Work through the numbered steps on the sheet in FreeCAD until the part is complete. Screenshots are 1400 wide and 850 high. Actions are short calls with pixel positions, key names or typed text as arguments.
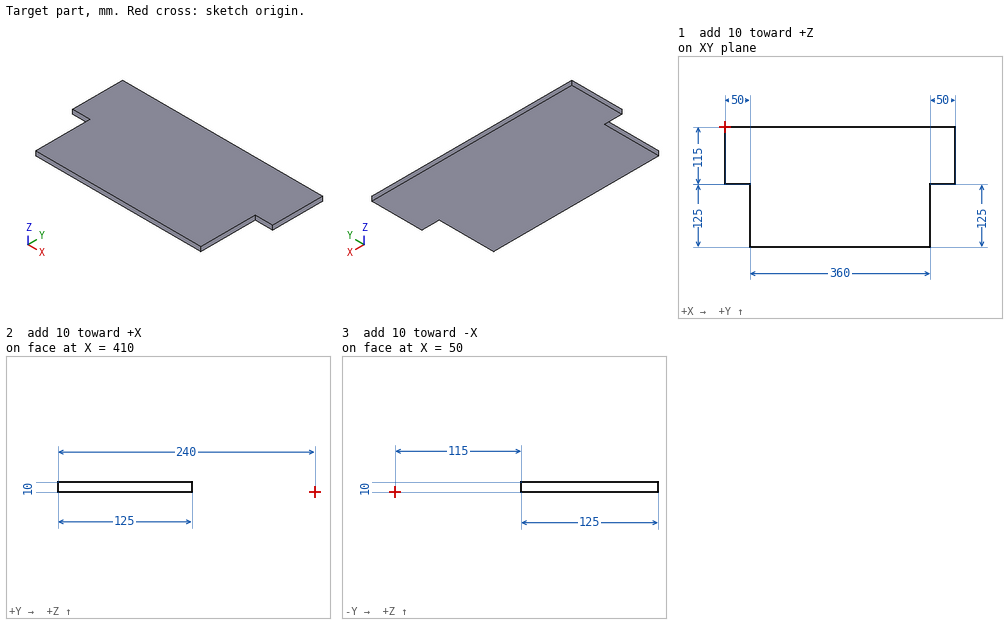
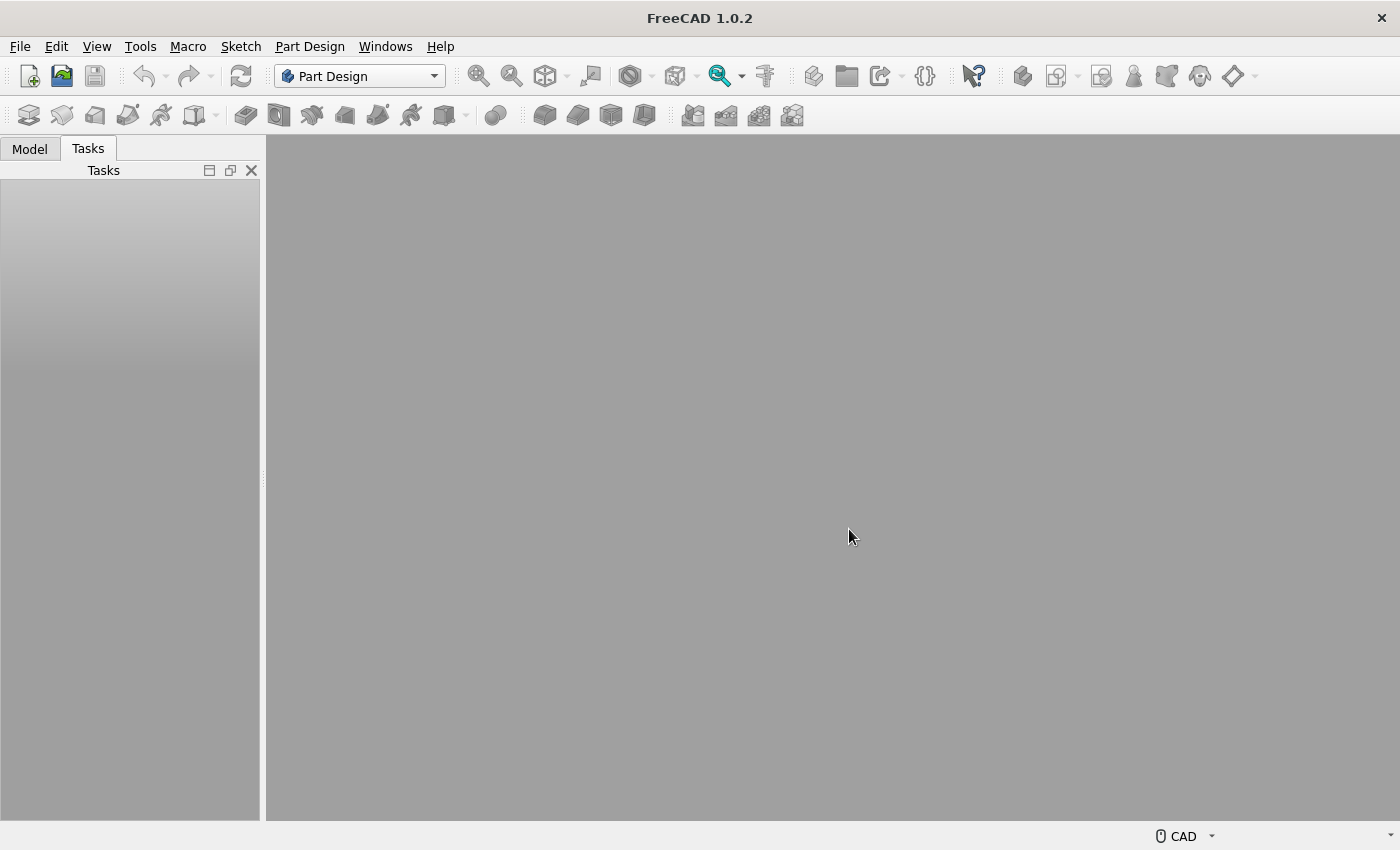
click(29, 76)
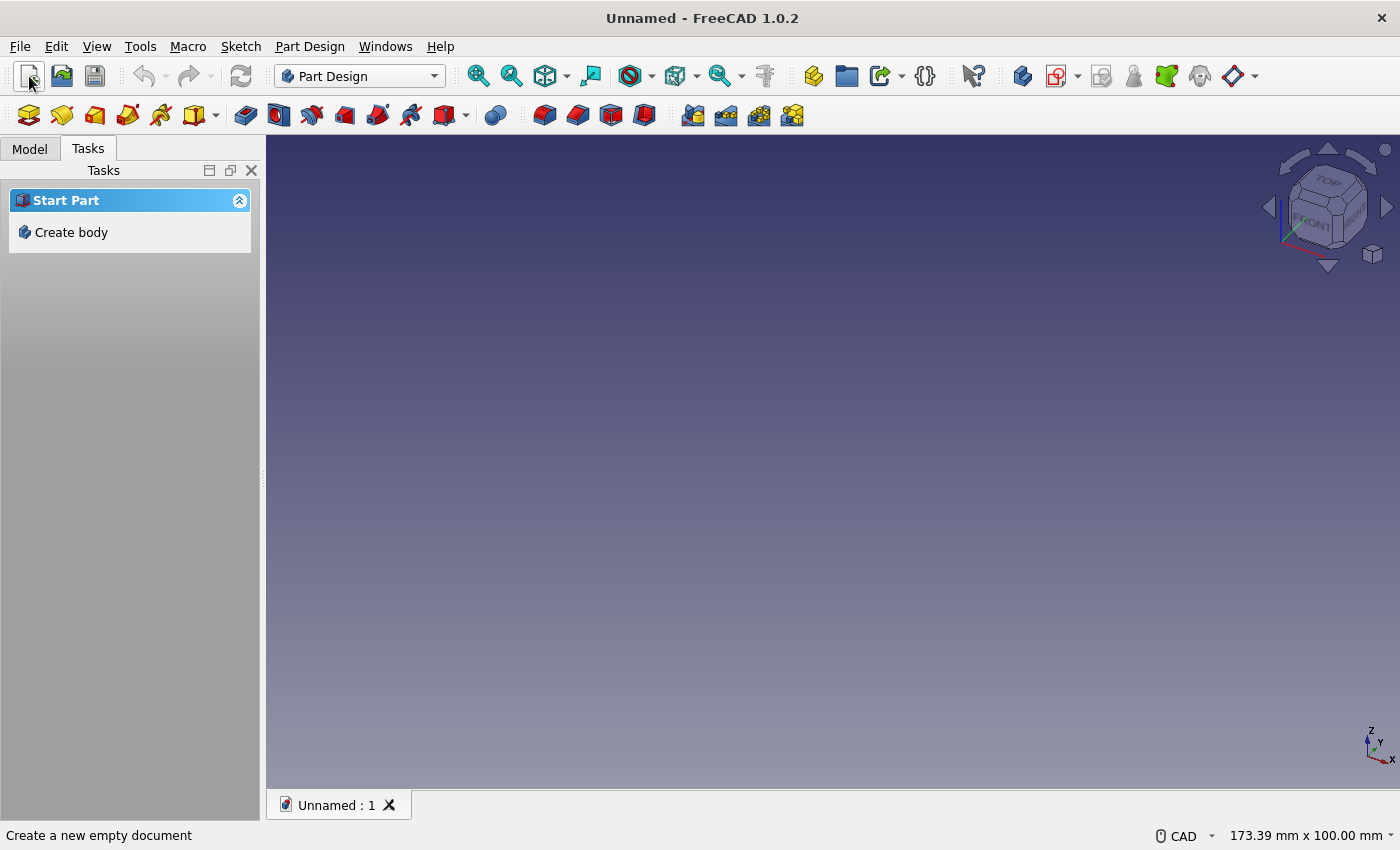
click(1056, 76)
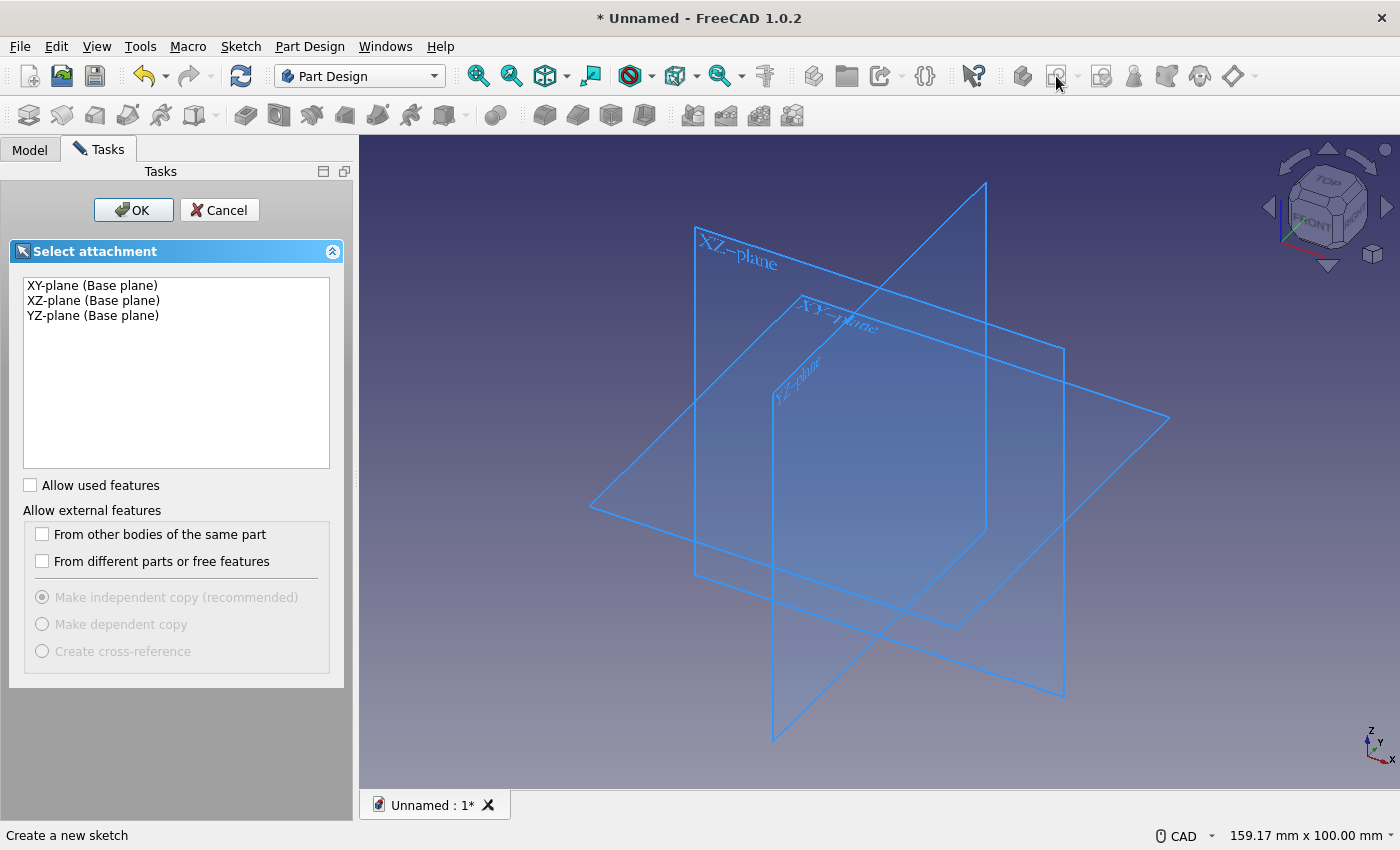
click(84, 286)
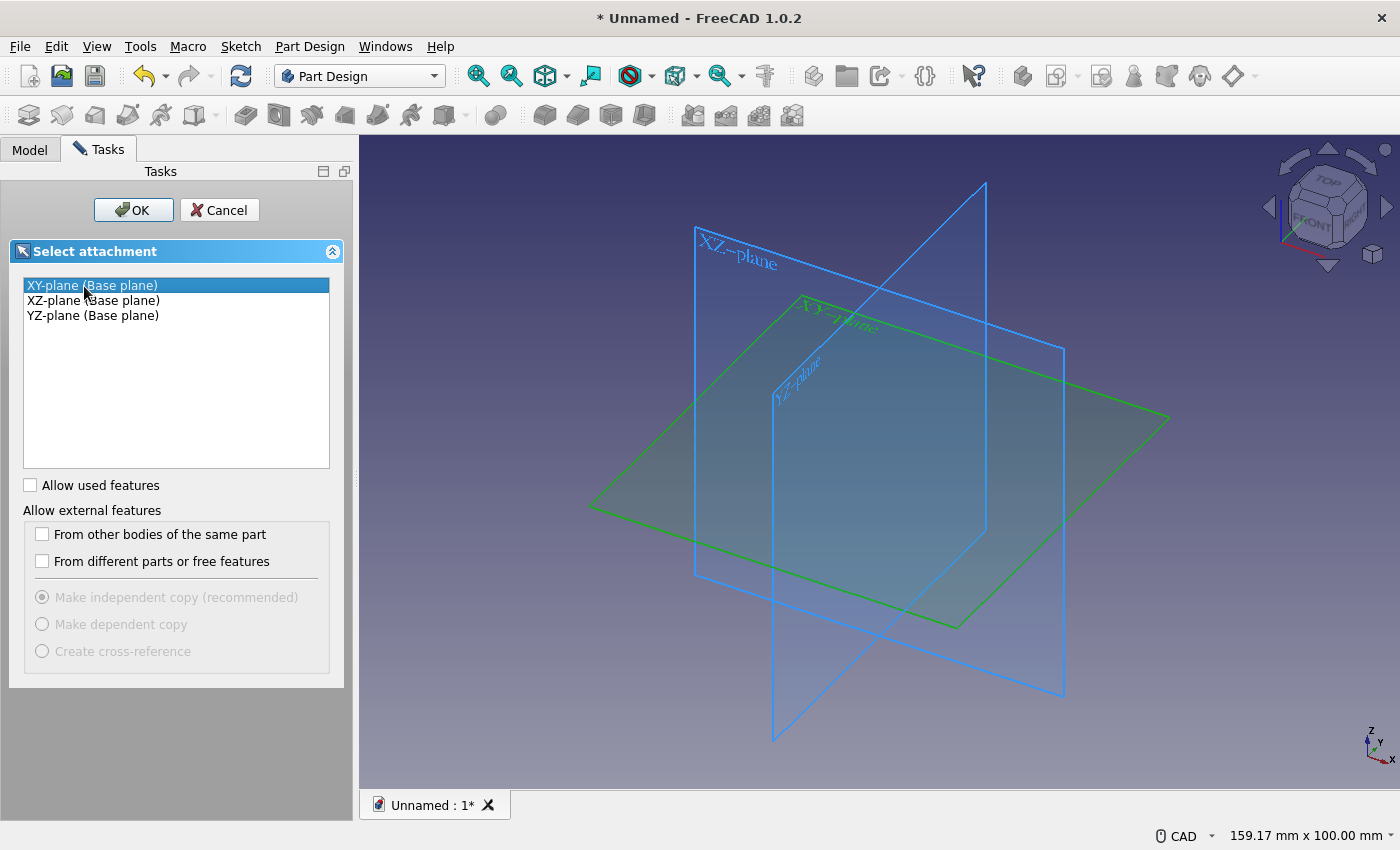
click(134, 210)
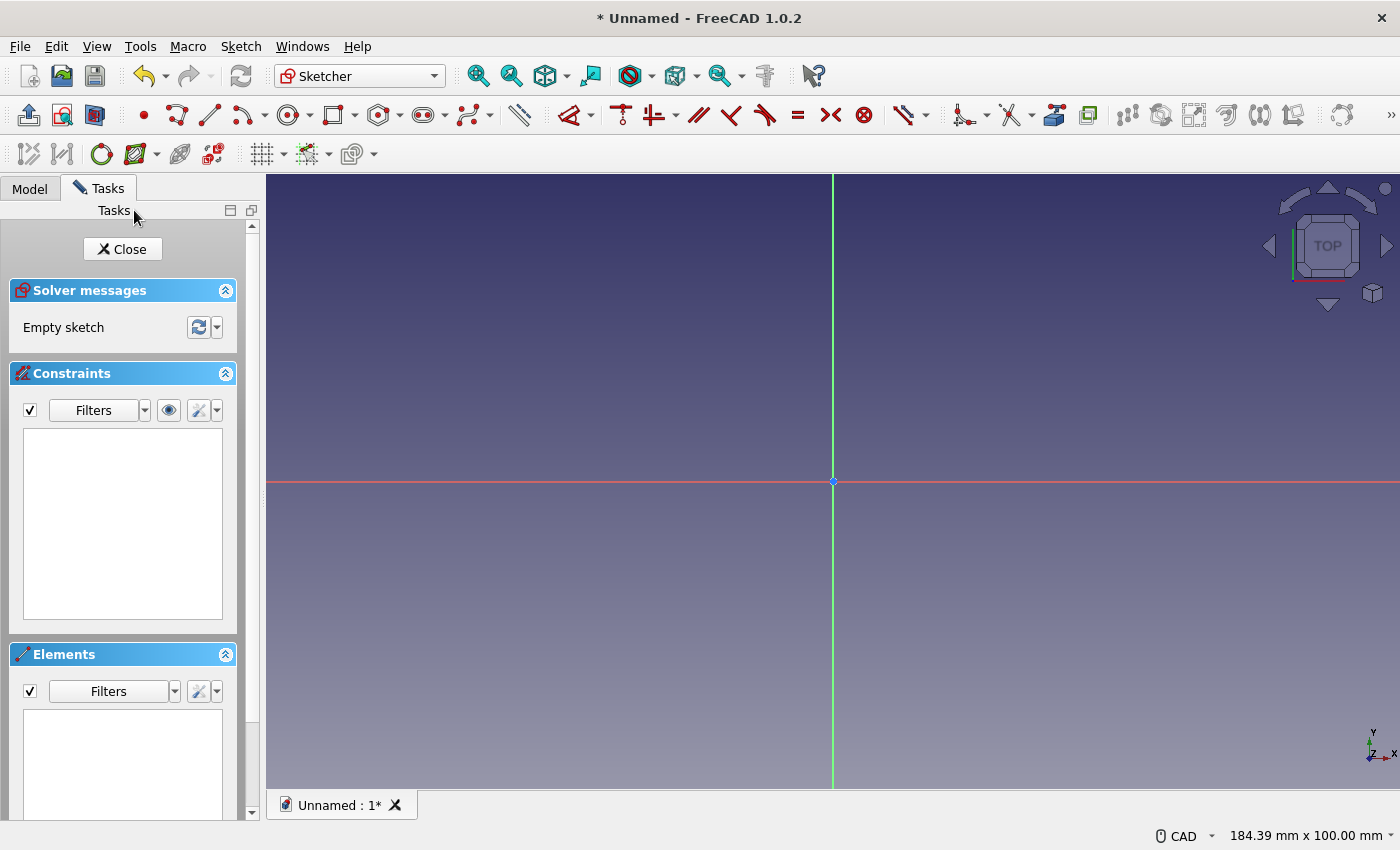
scroll(294, 240, down, 7)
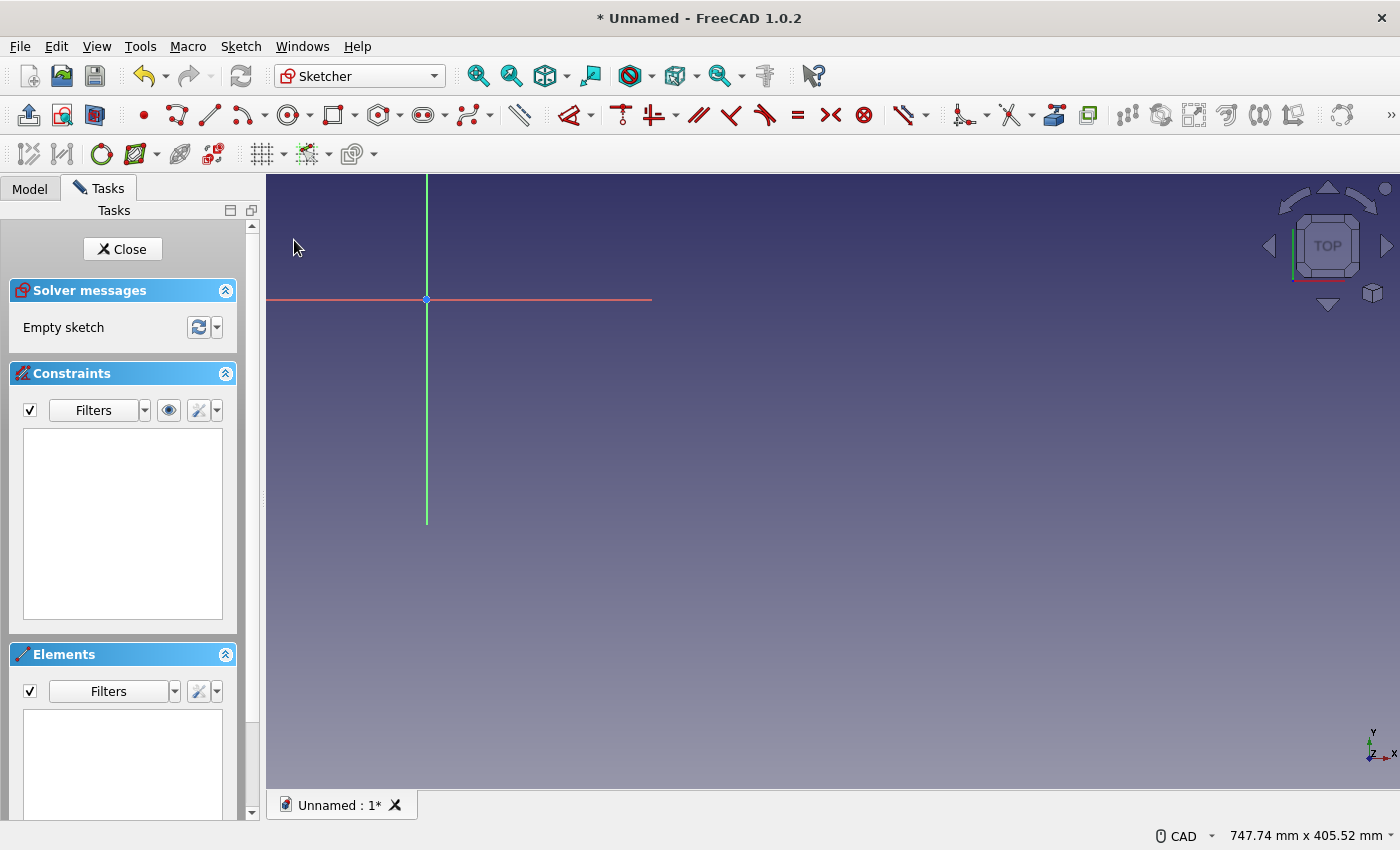
click(177, 116)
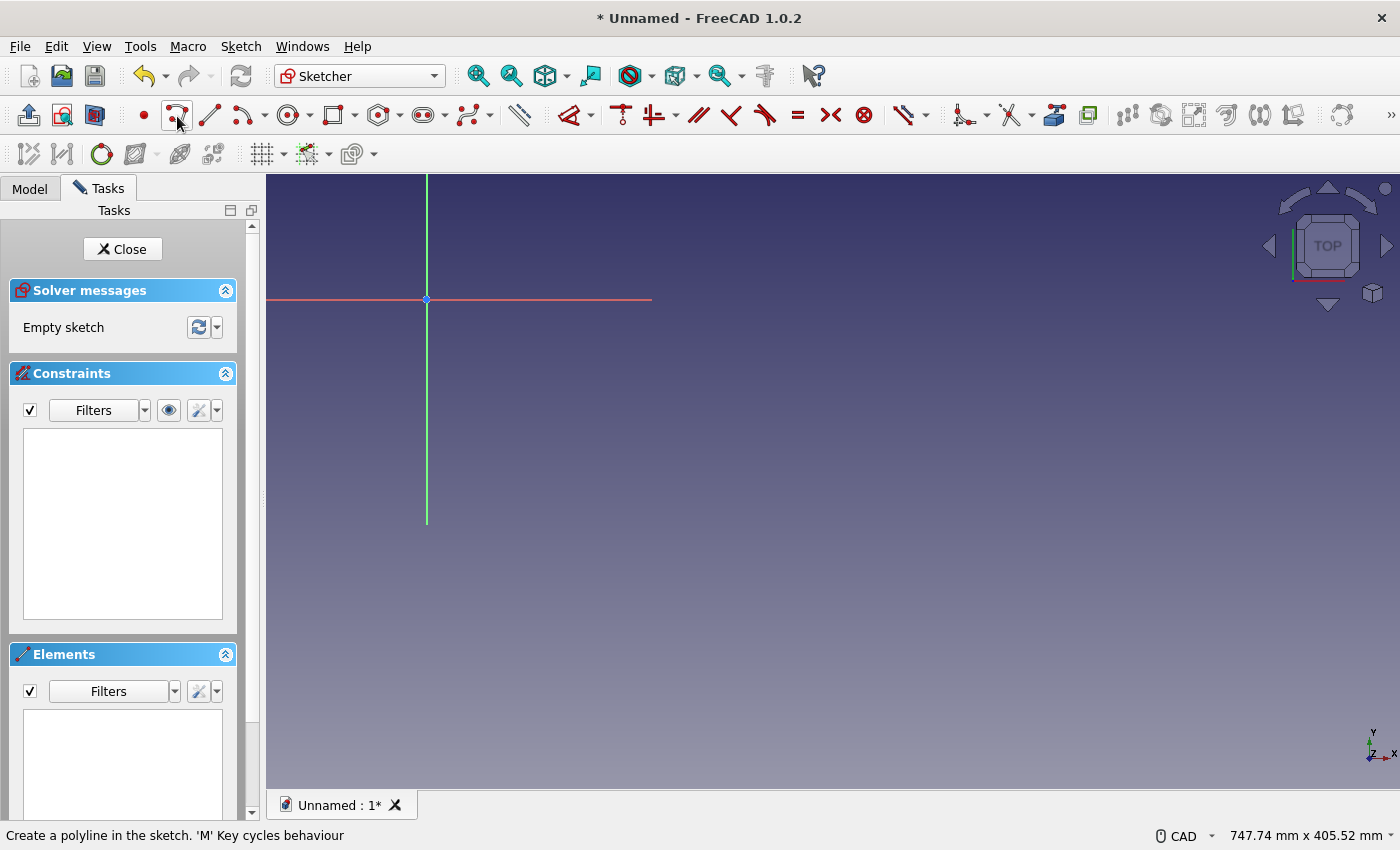
click(427, 300)
click(436, 474)
click(503, 474)
click(503, 664)
click(1049, 664)
click(1049, 474)
click(1125, 474)
click(1125, 309)
click(427, 300)
key(Escape)
key(Escape)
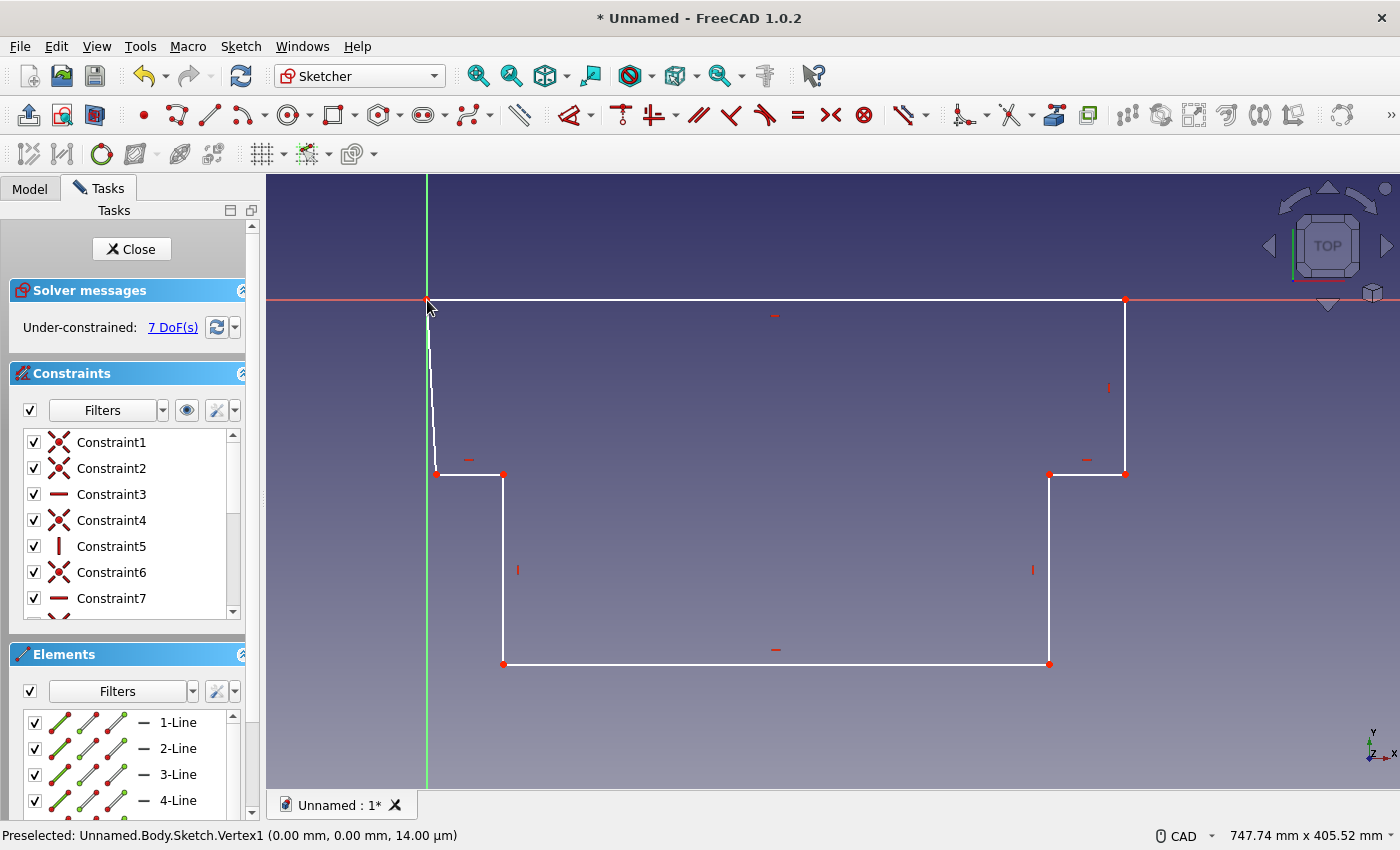
click(430, 352)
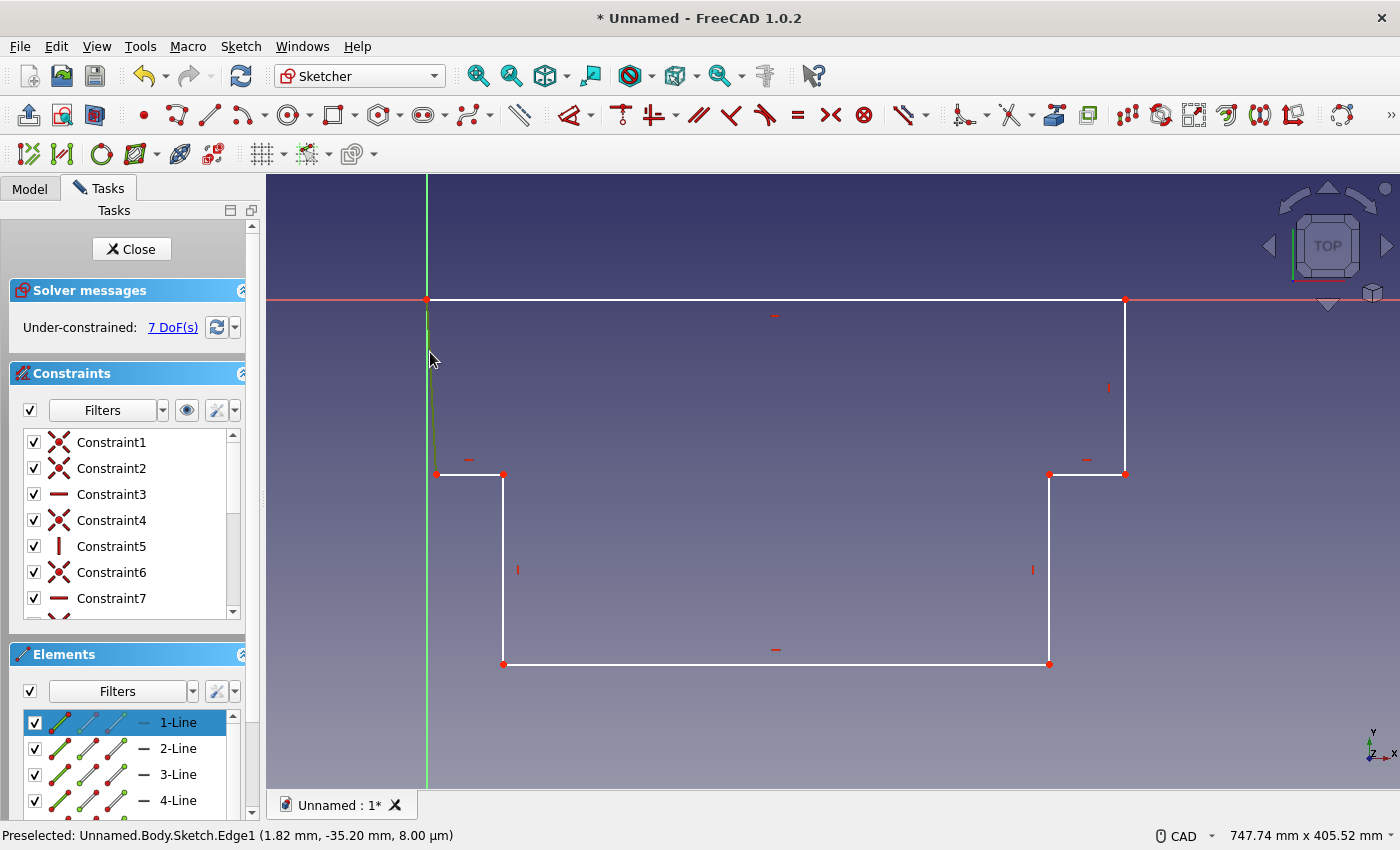
click(676, 116)